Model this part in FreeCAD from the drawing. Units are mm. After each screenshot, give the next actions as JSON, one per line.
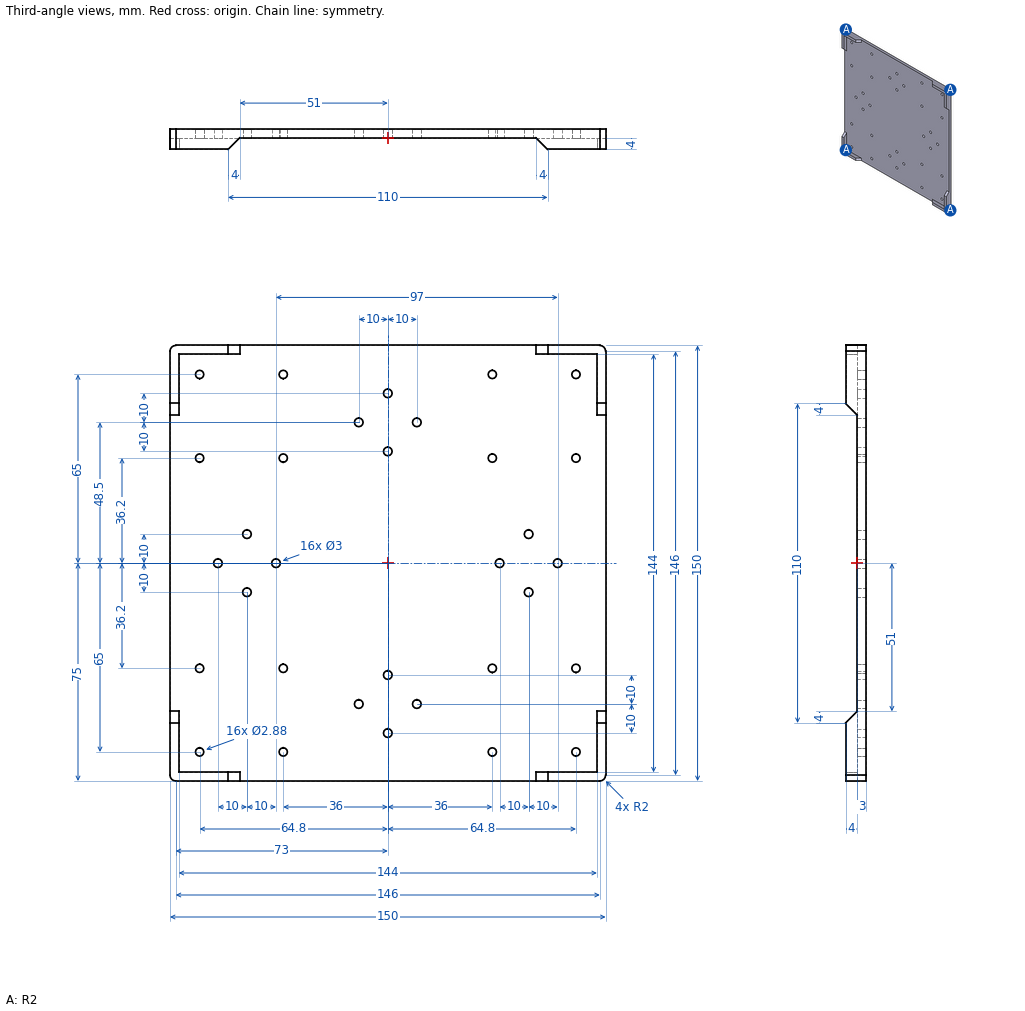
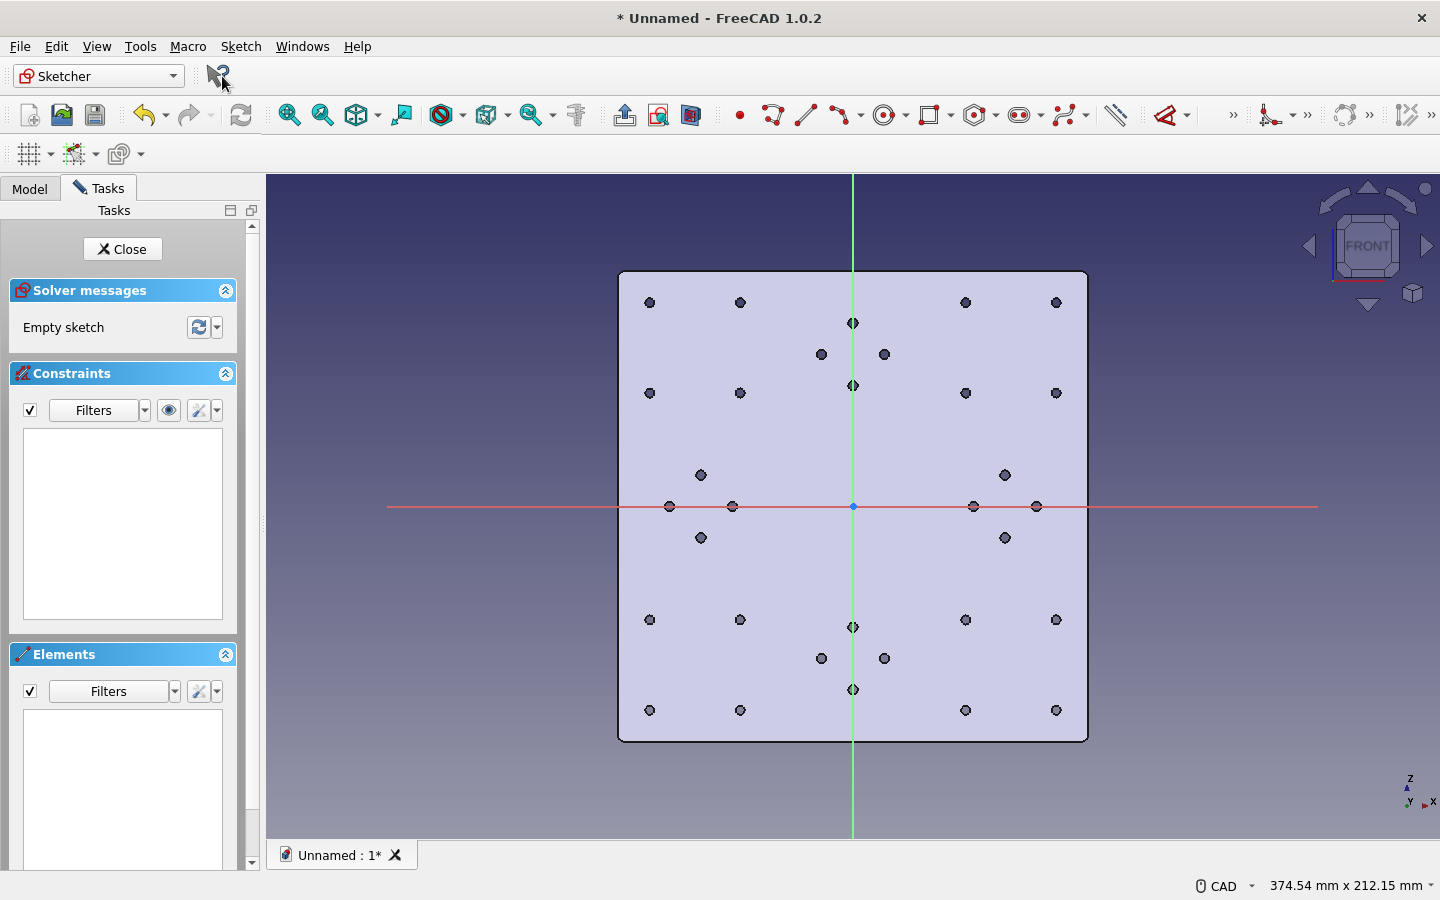
{"action": "key", "text": "g l"}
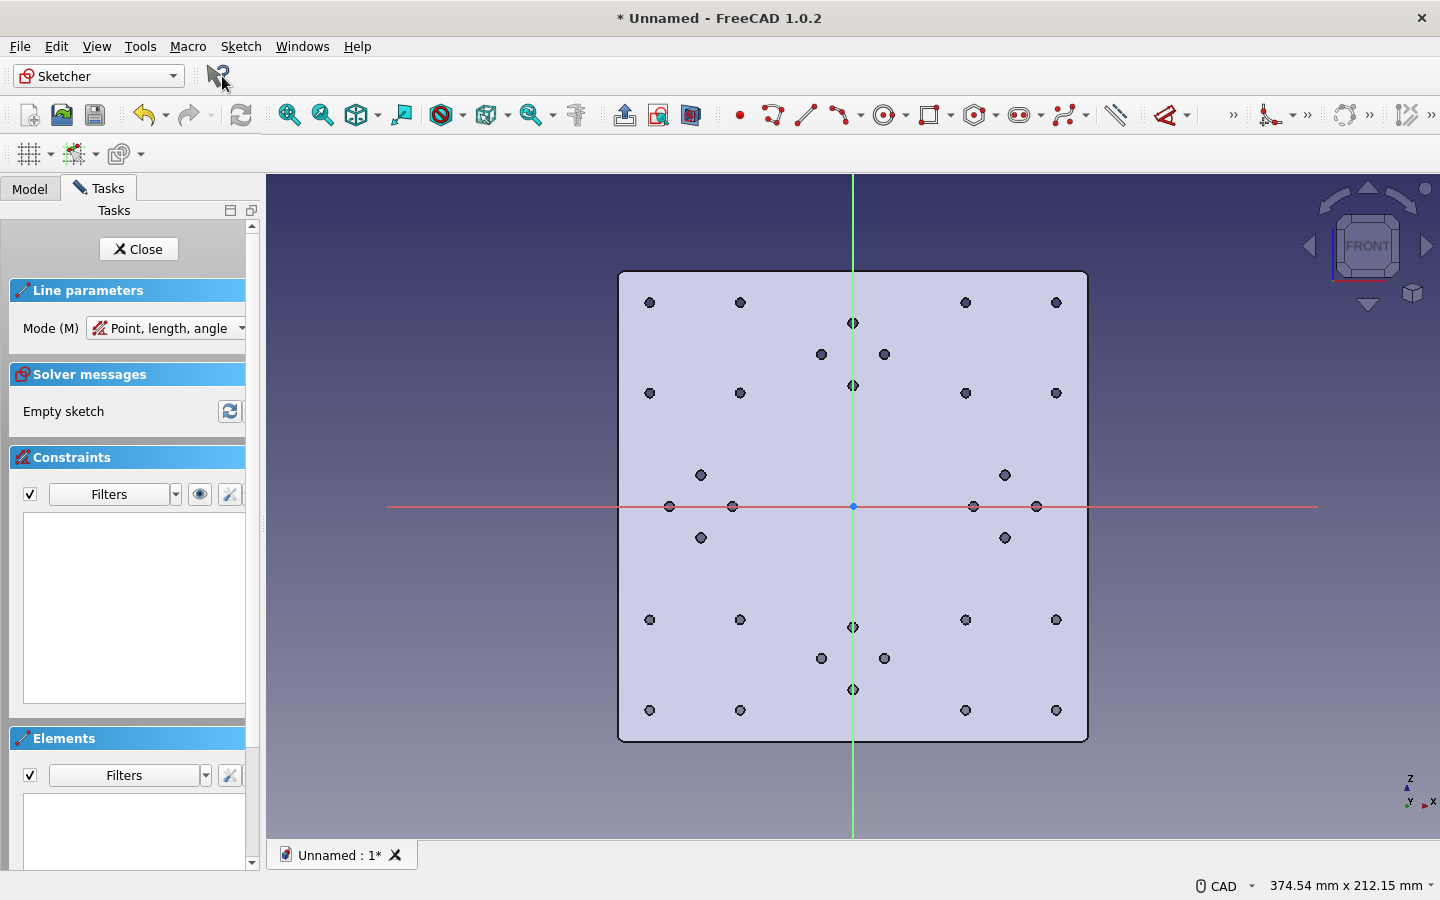
{"action": "left_click", "coordinate": [624, 742]}
{"action": "left_click", "coordinate": [1082, 742]}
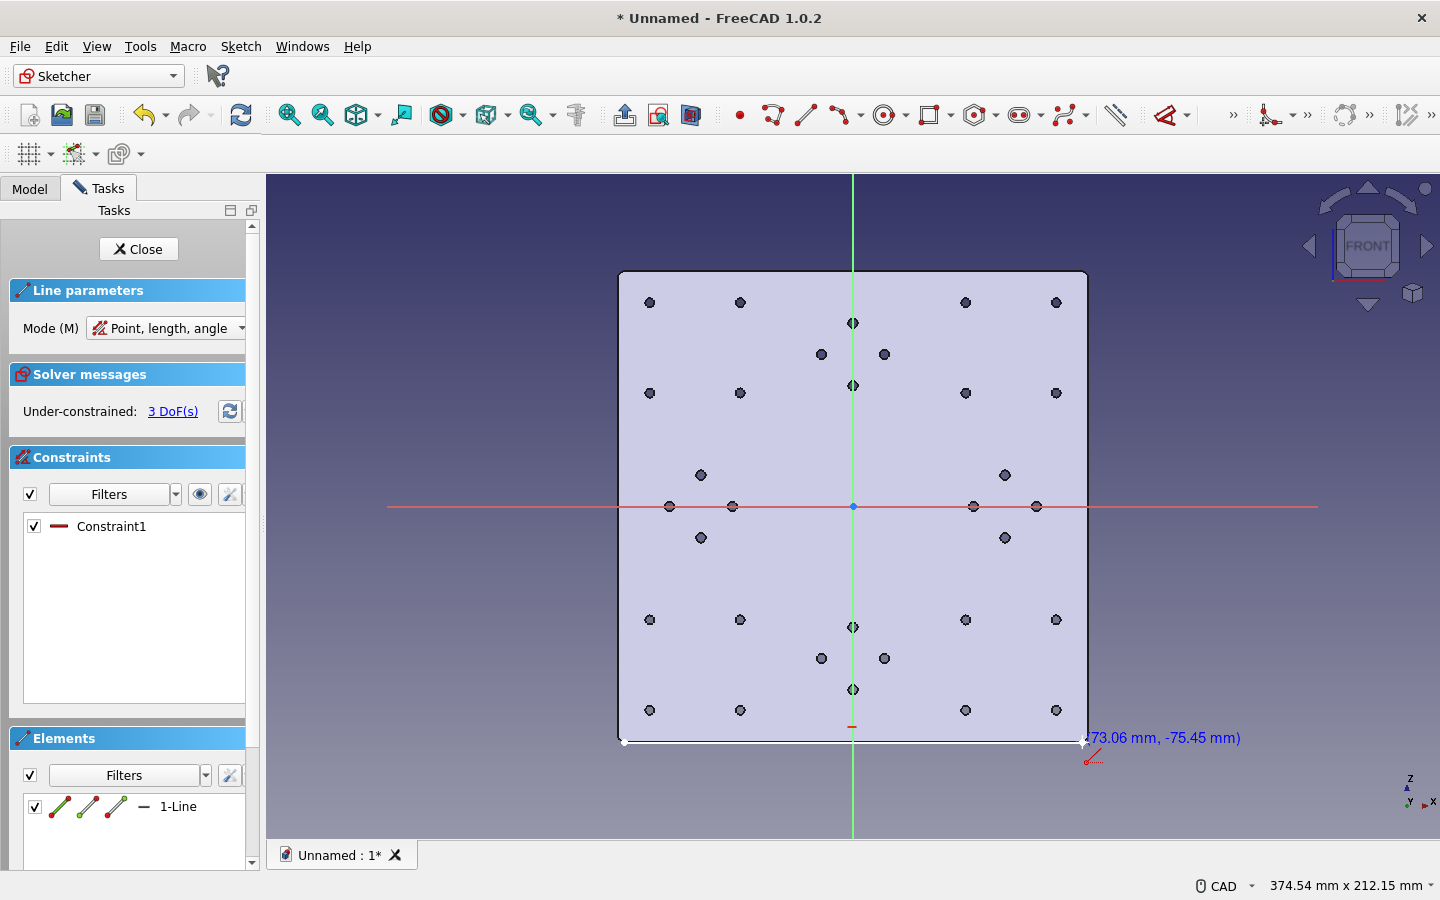
{"action": "scroll", "coordinate": [1088, 735], "scroll_direction": "up", "scroll_amount": 3}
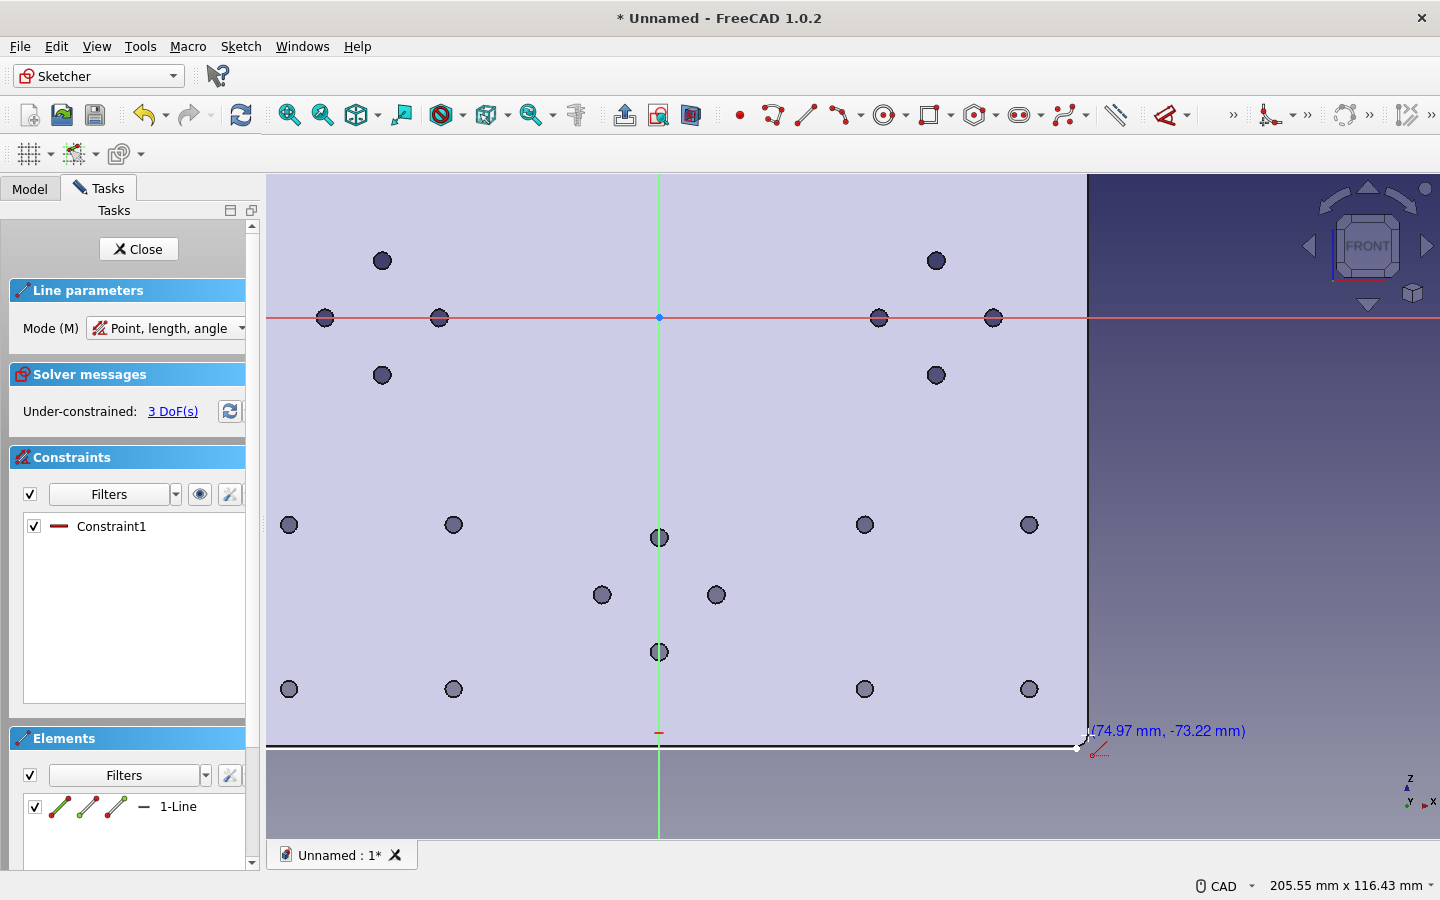
{"action": "left_click", "coordinate": [1088, 735]}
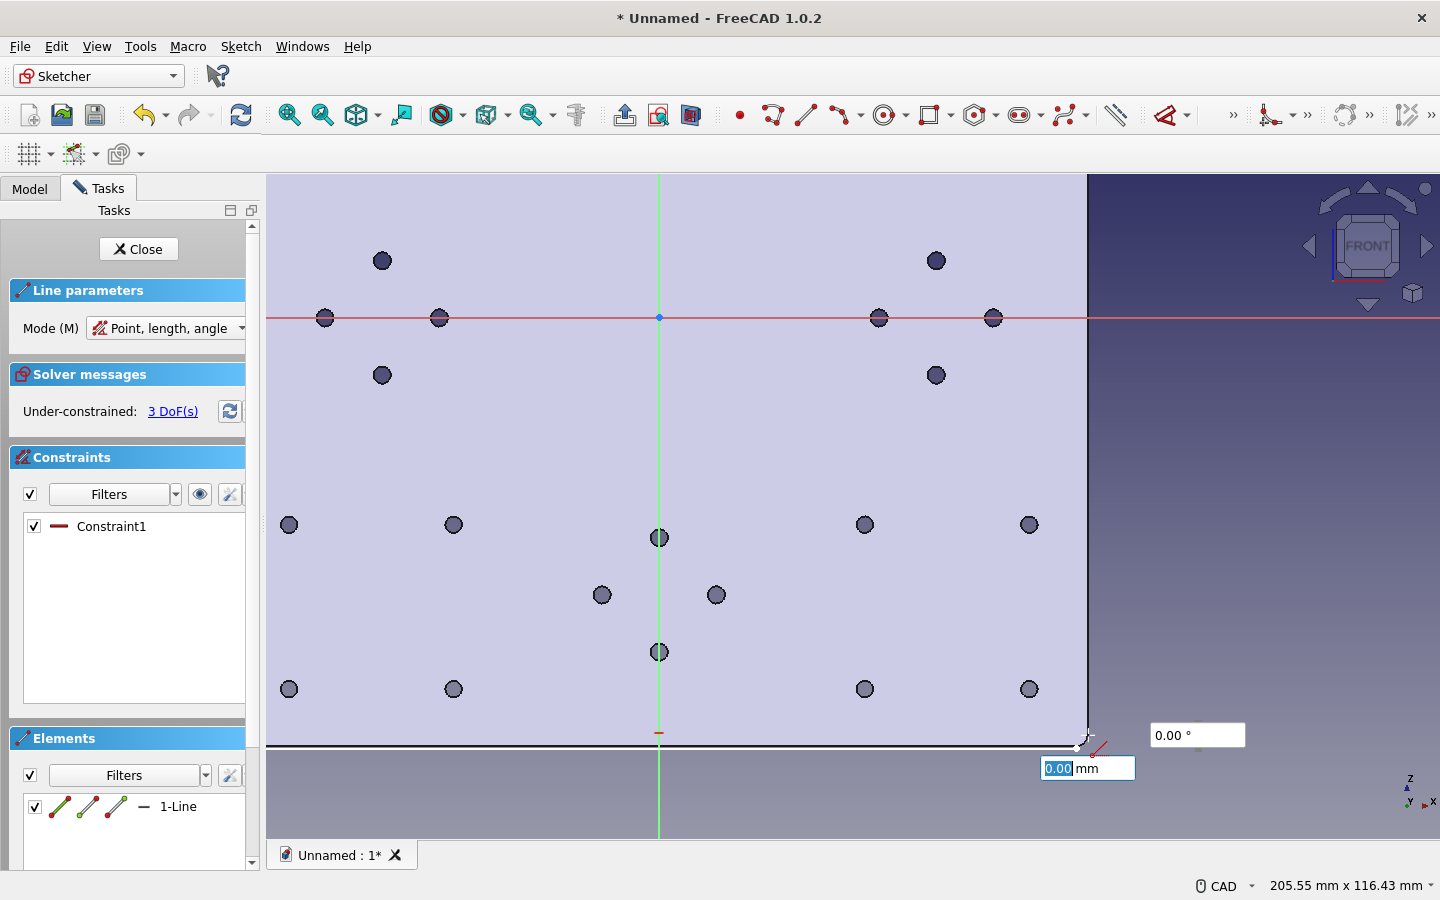
{"action": "scroll", "coordinate": [937, 736], "scroll_direction": "down", "scroll_amount": 3}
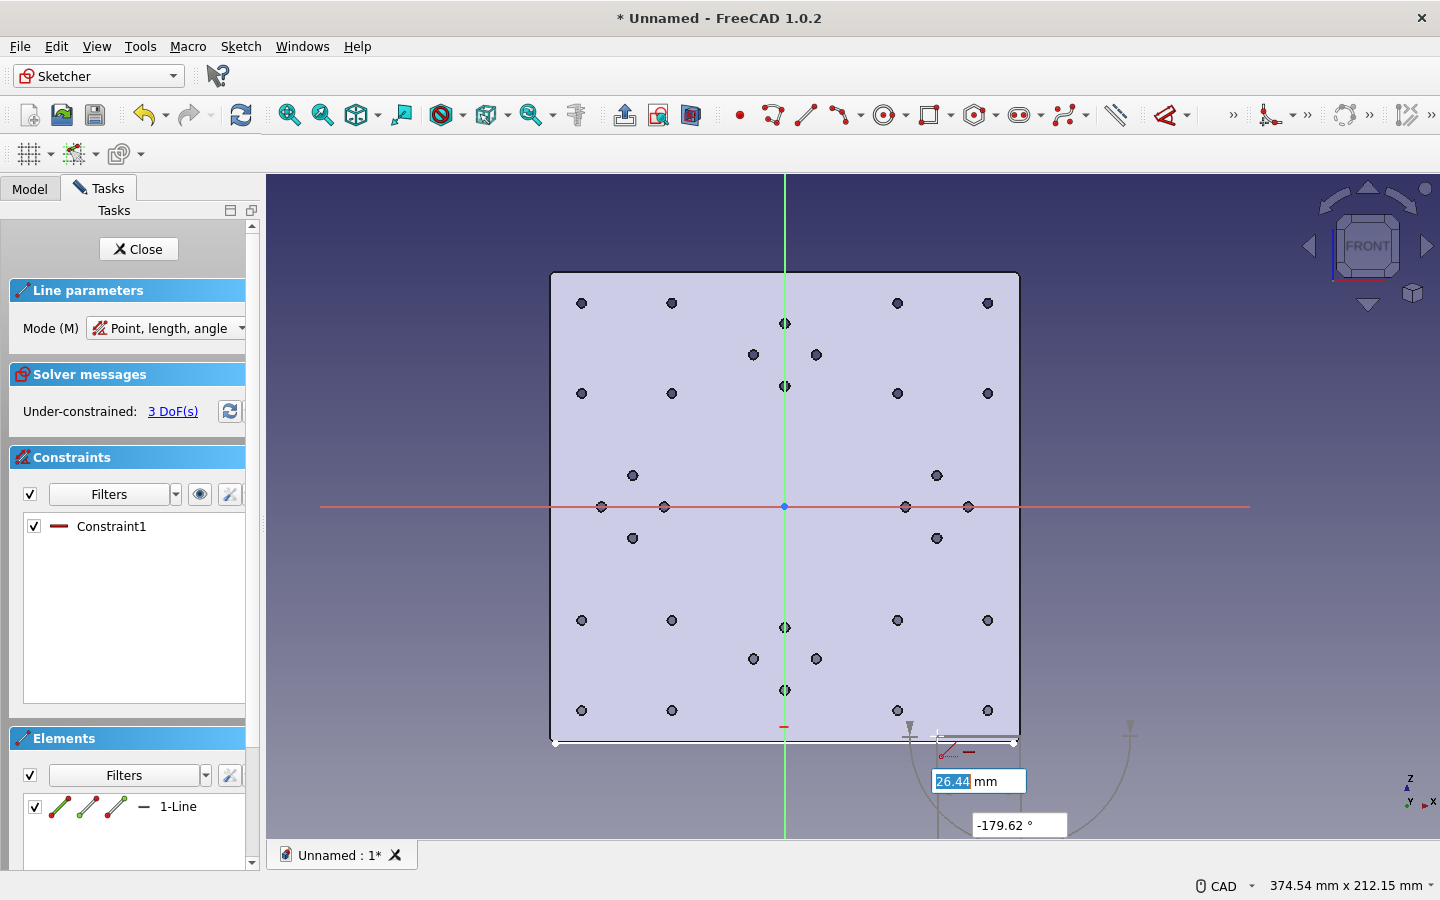
{"action": "left_click", "coordinate": [1020, 278]}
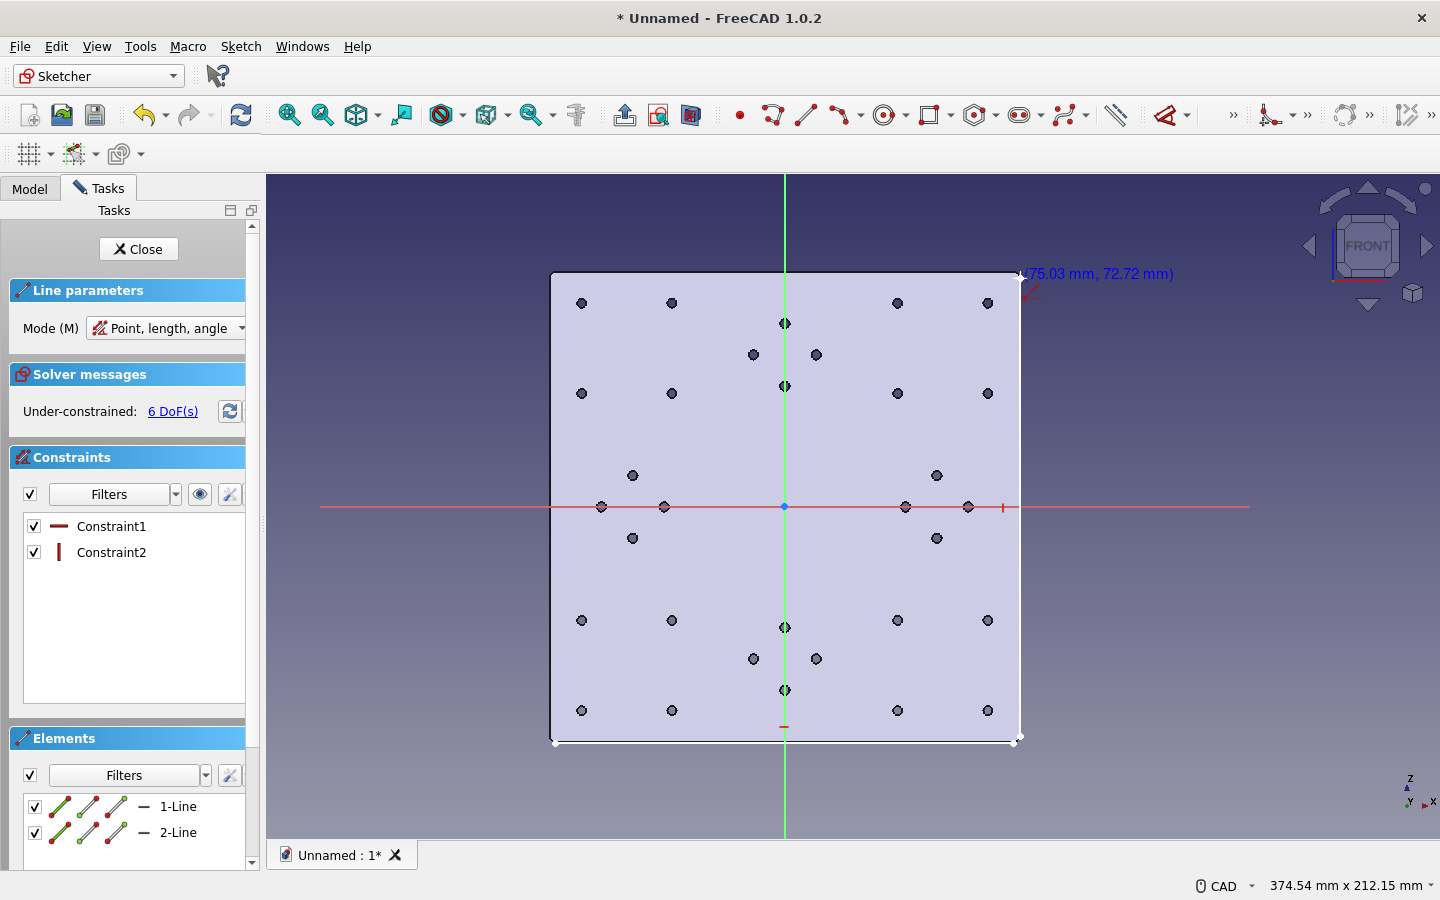
{"action": "scroll", "coordinate": [1014, 272], "scroll_direction": "up", "scroll_amount": 3}